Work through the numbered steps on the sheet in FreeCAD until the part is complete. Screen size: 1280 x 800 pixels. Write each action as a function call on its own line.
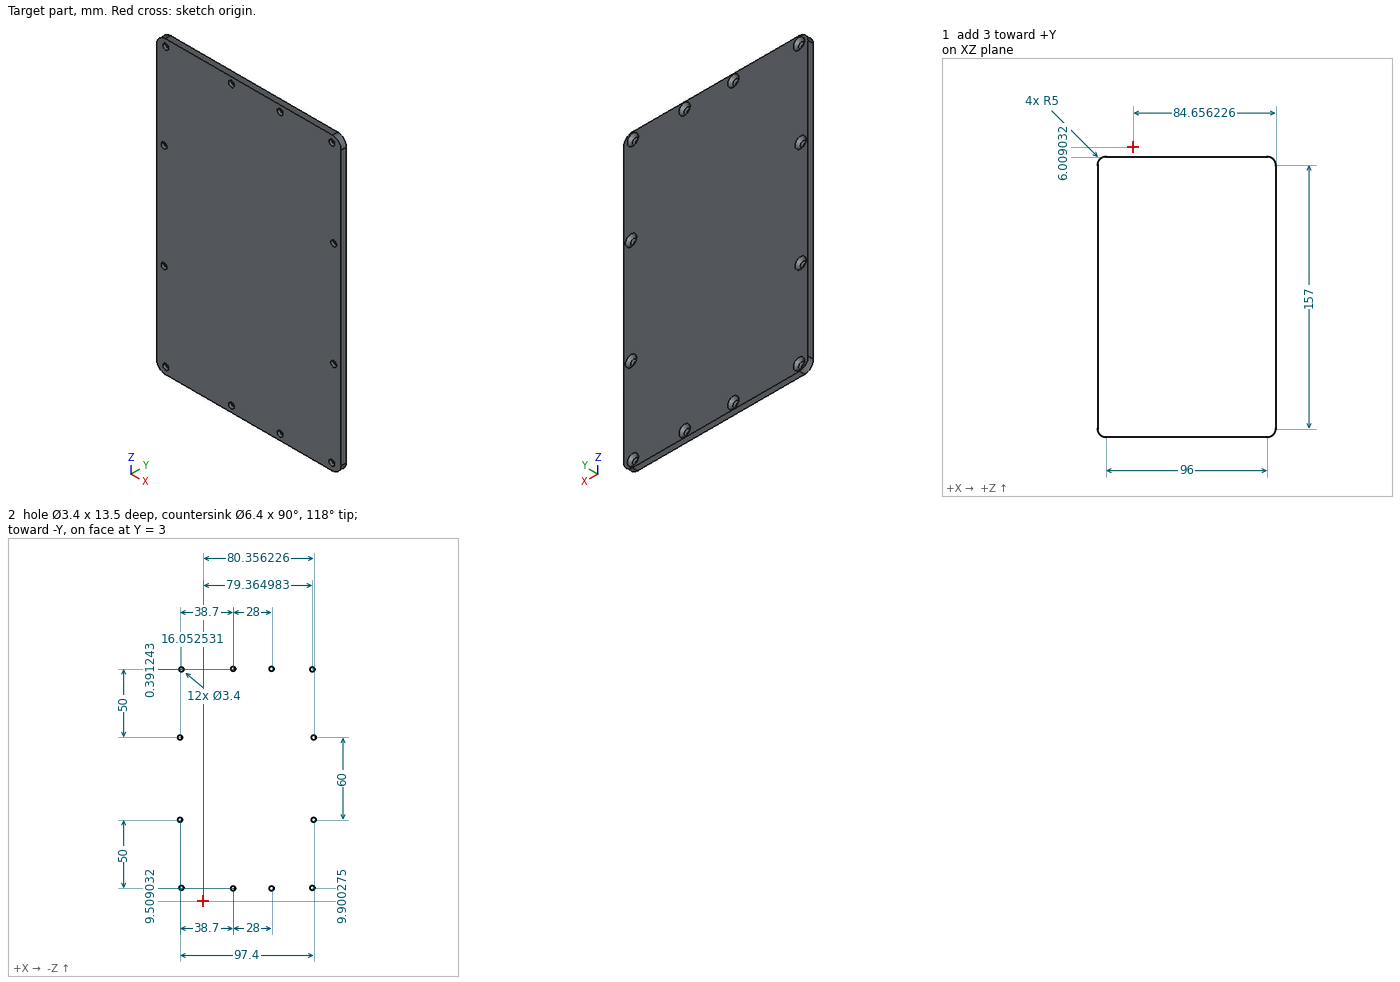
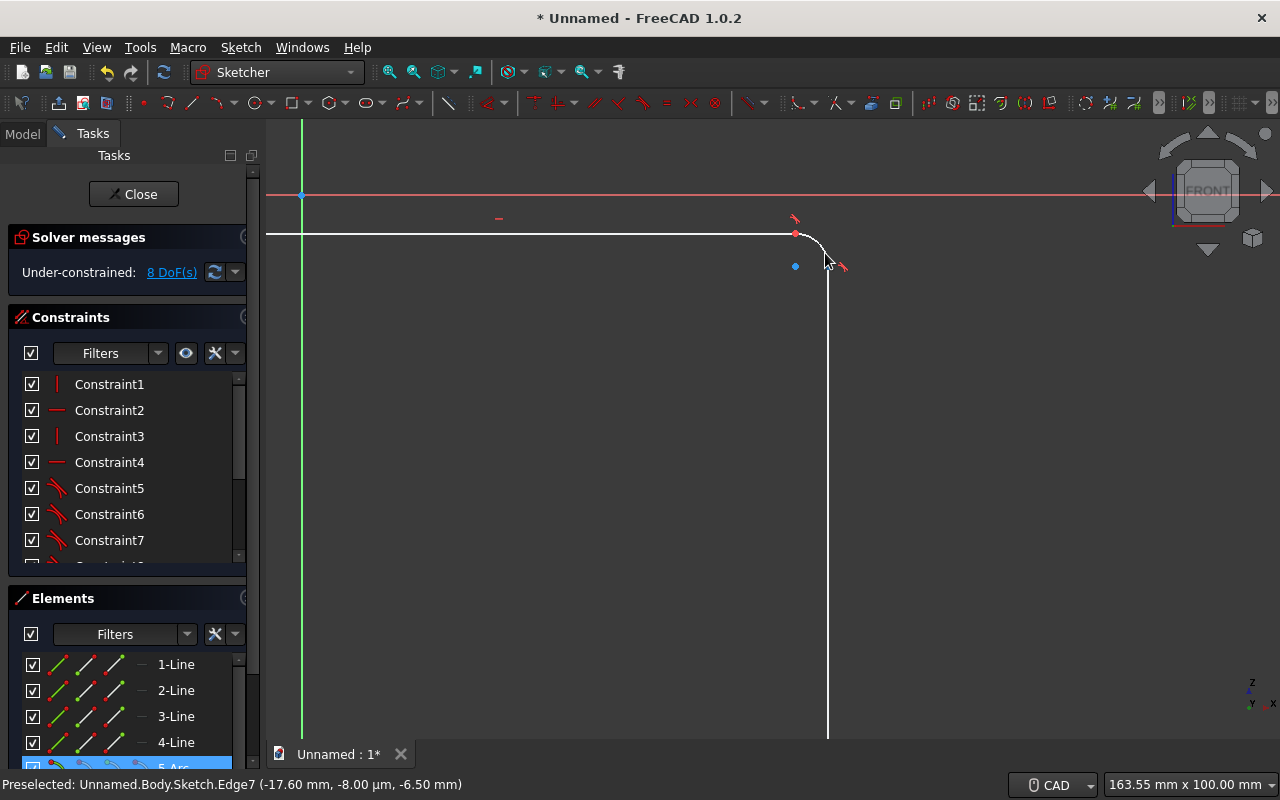
click(825, 252)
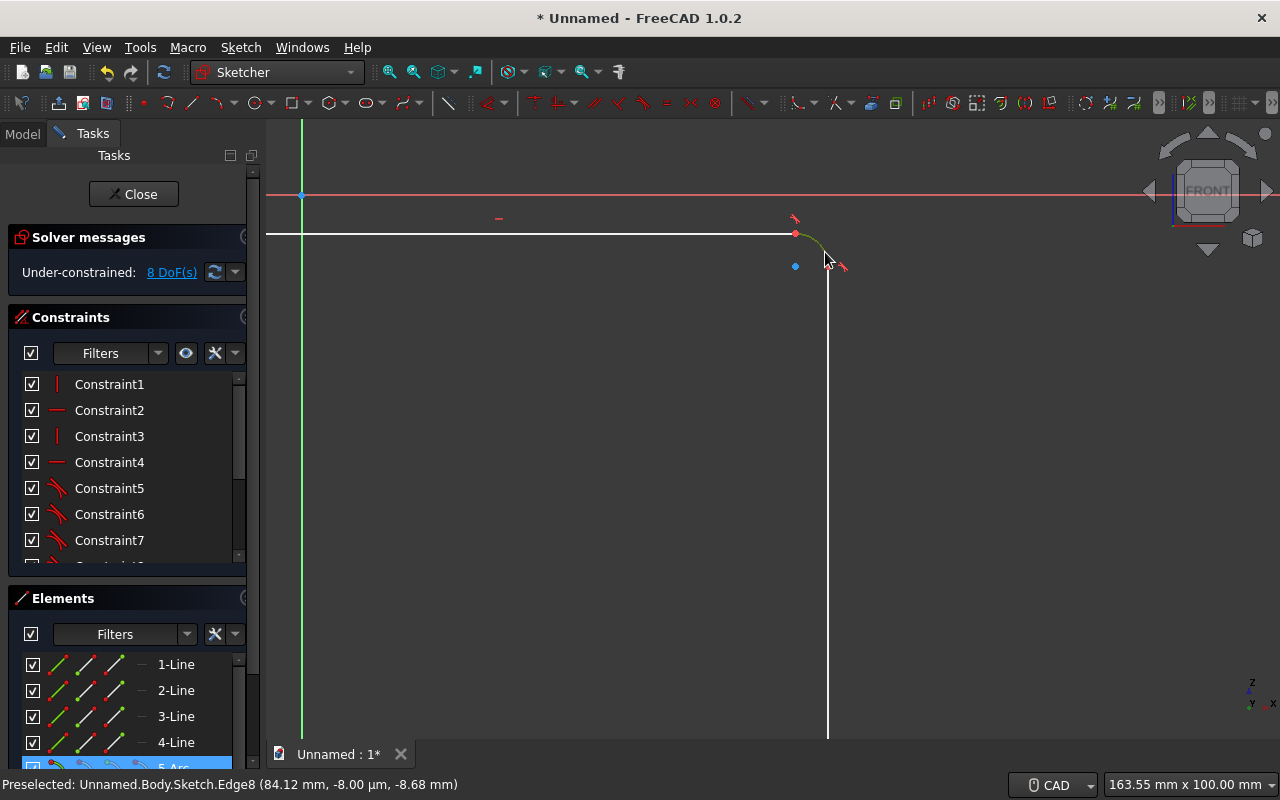
click(668, 104)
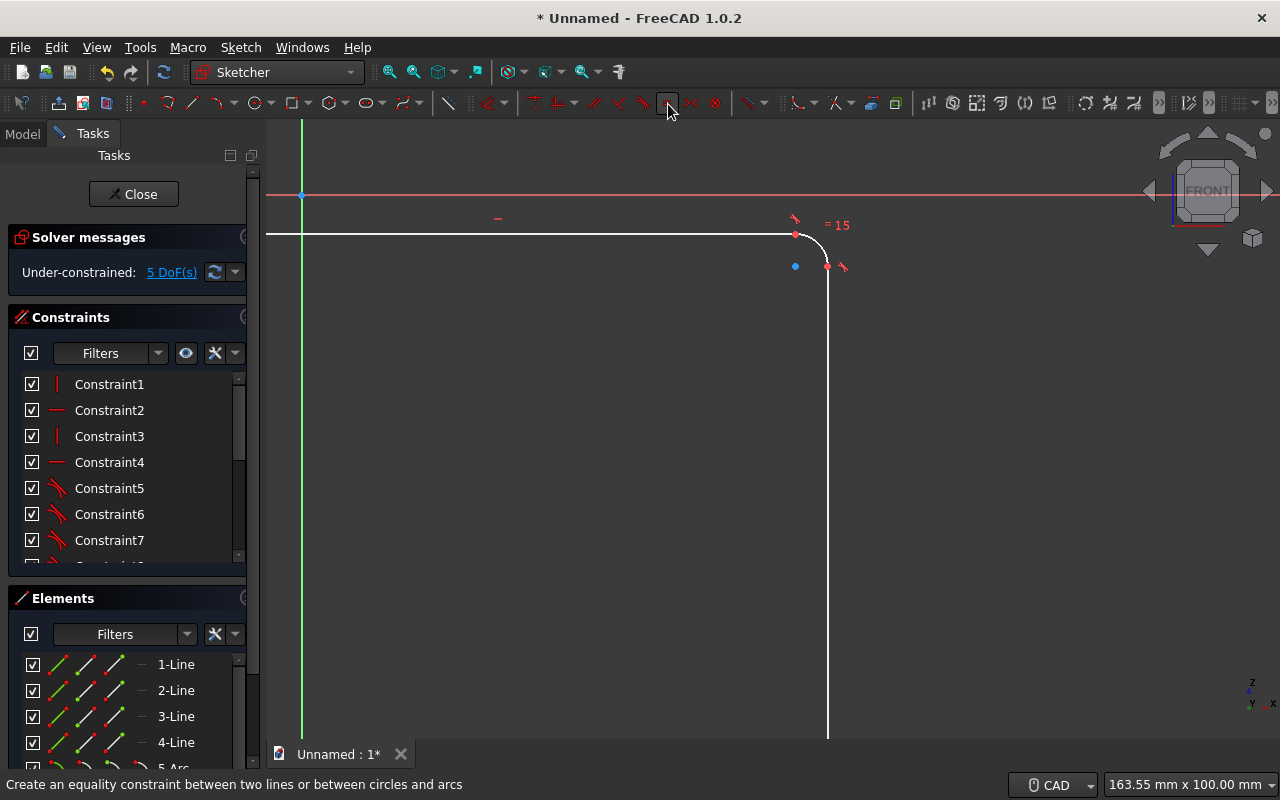
click(488, 104)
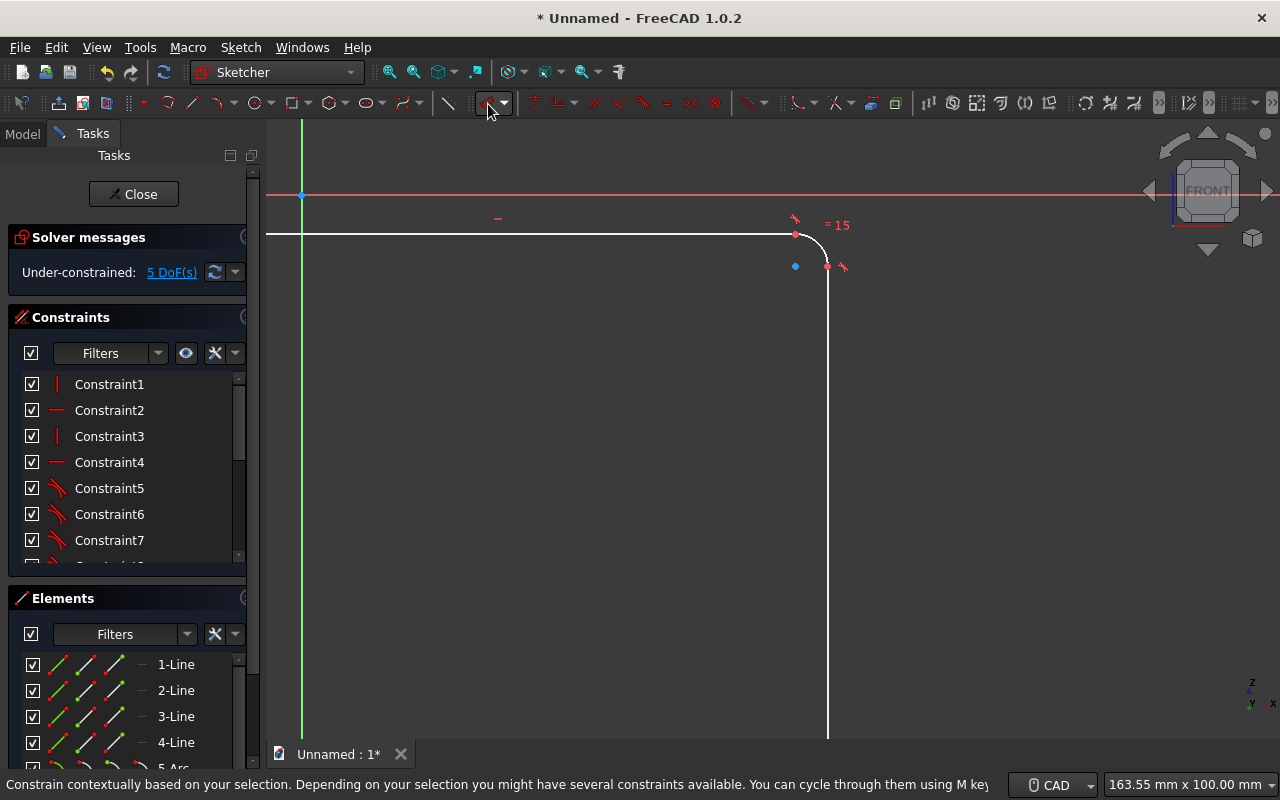
scroll(825, 253, down, 5)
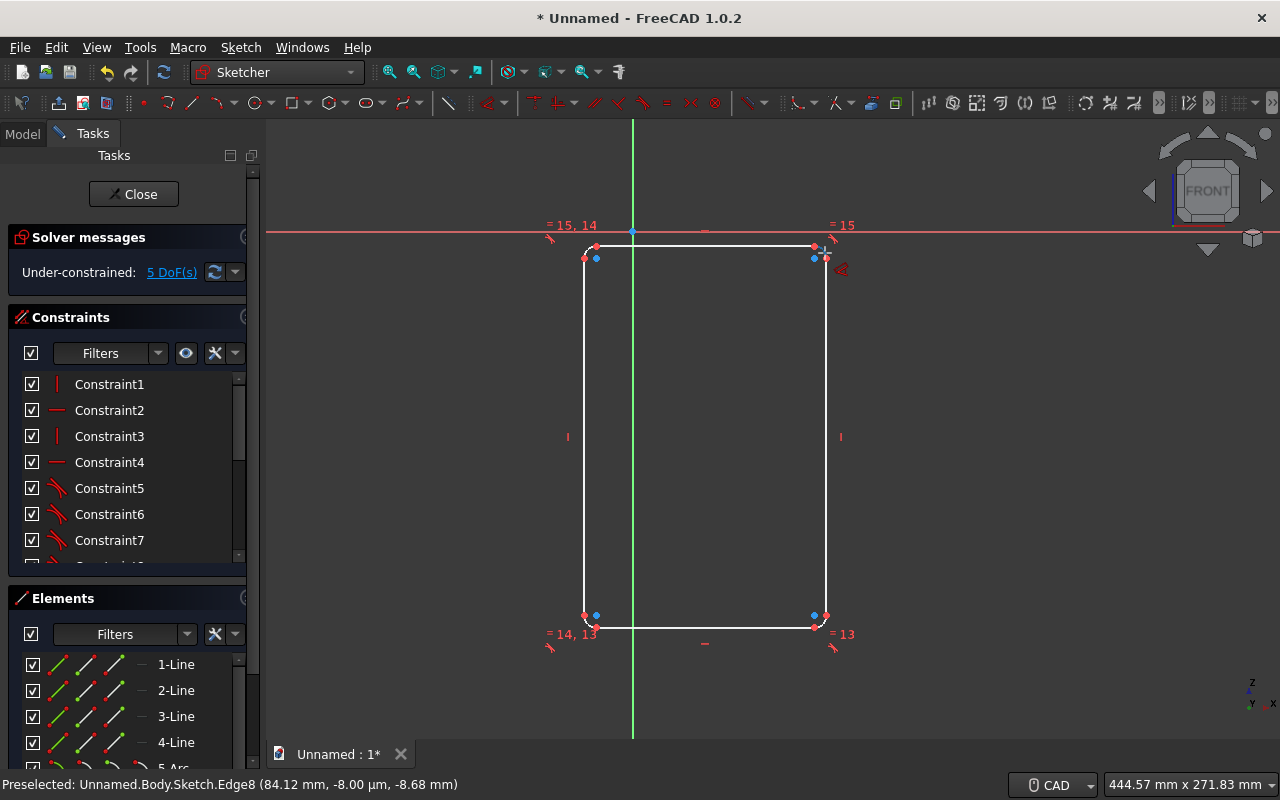
scroll(820, 627, up, 7)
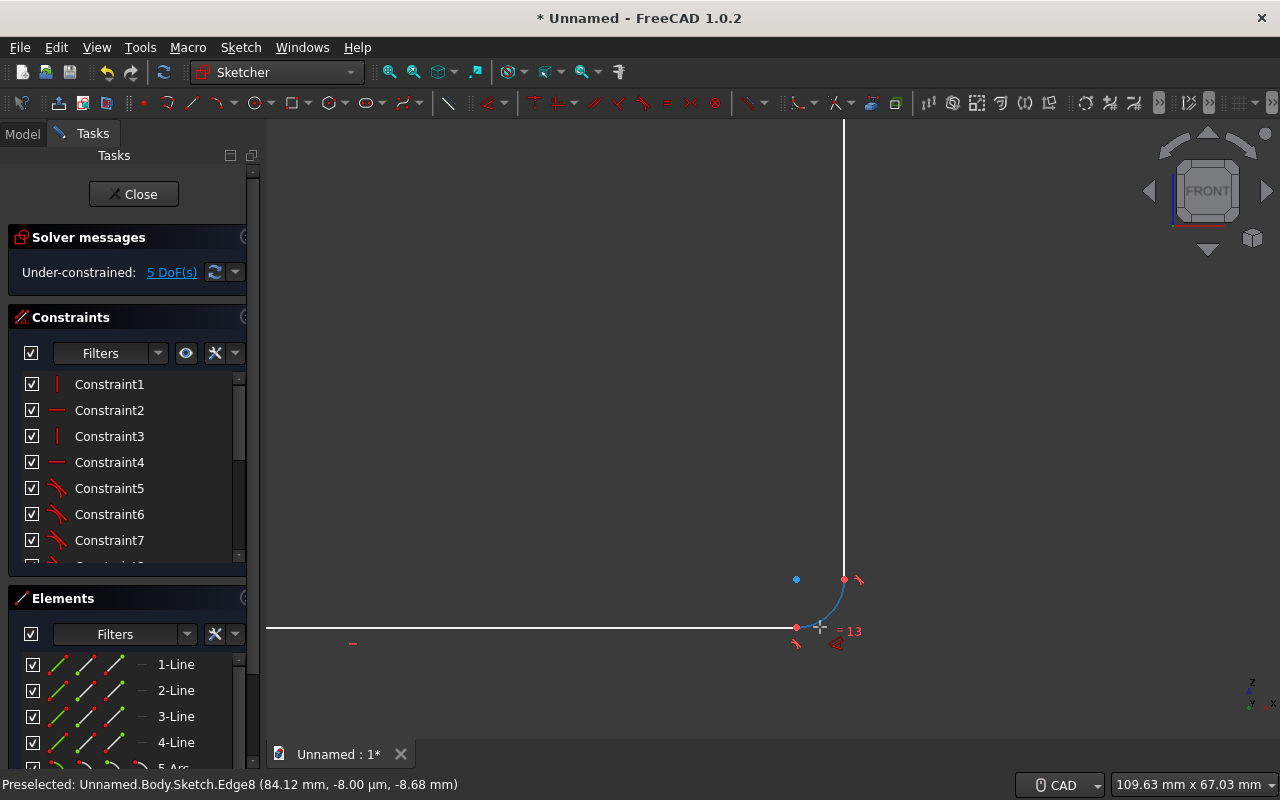
click(818, 623)
click(832, 652)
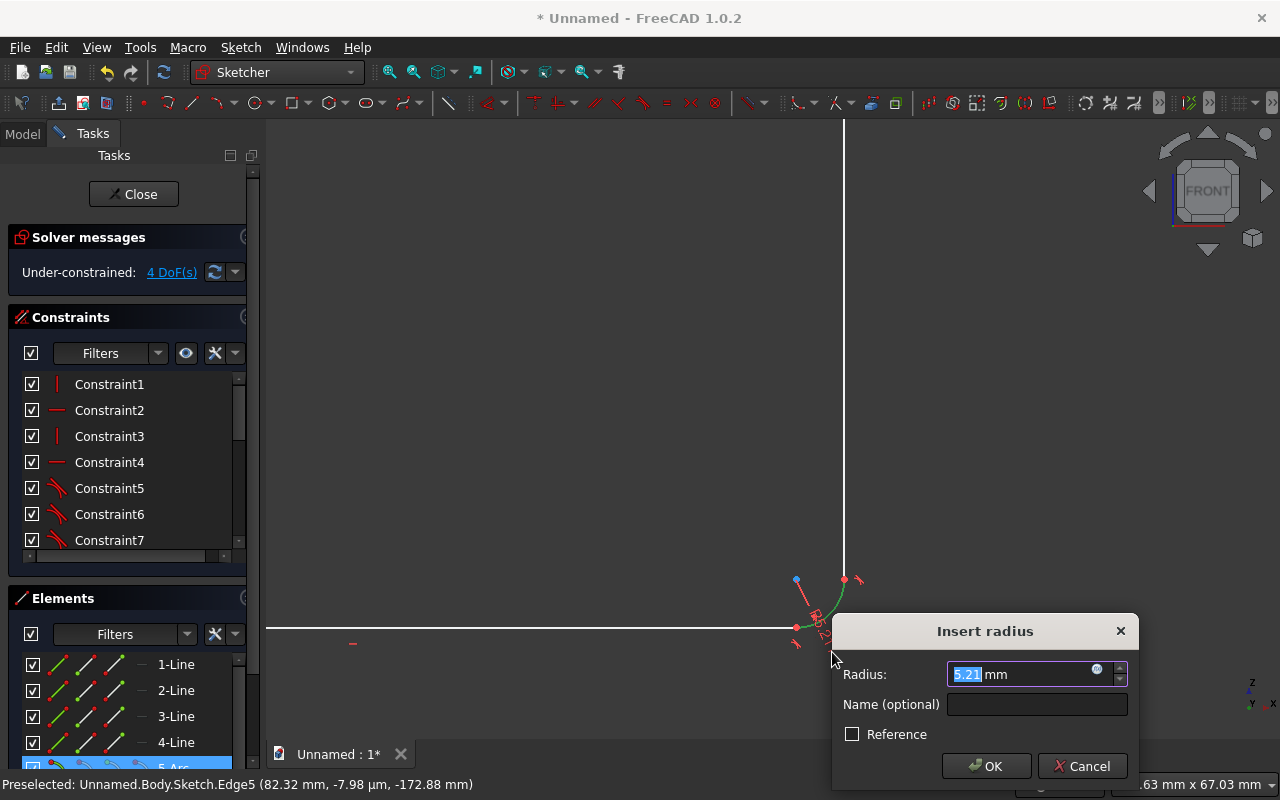
text(5)
key(Return)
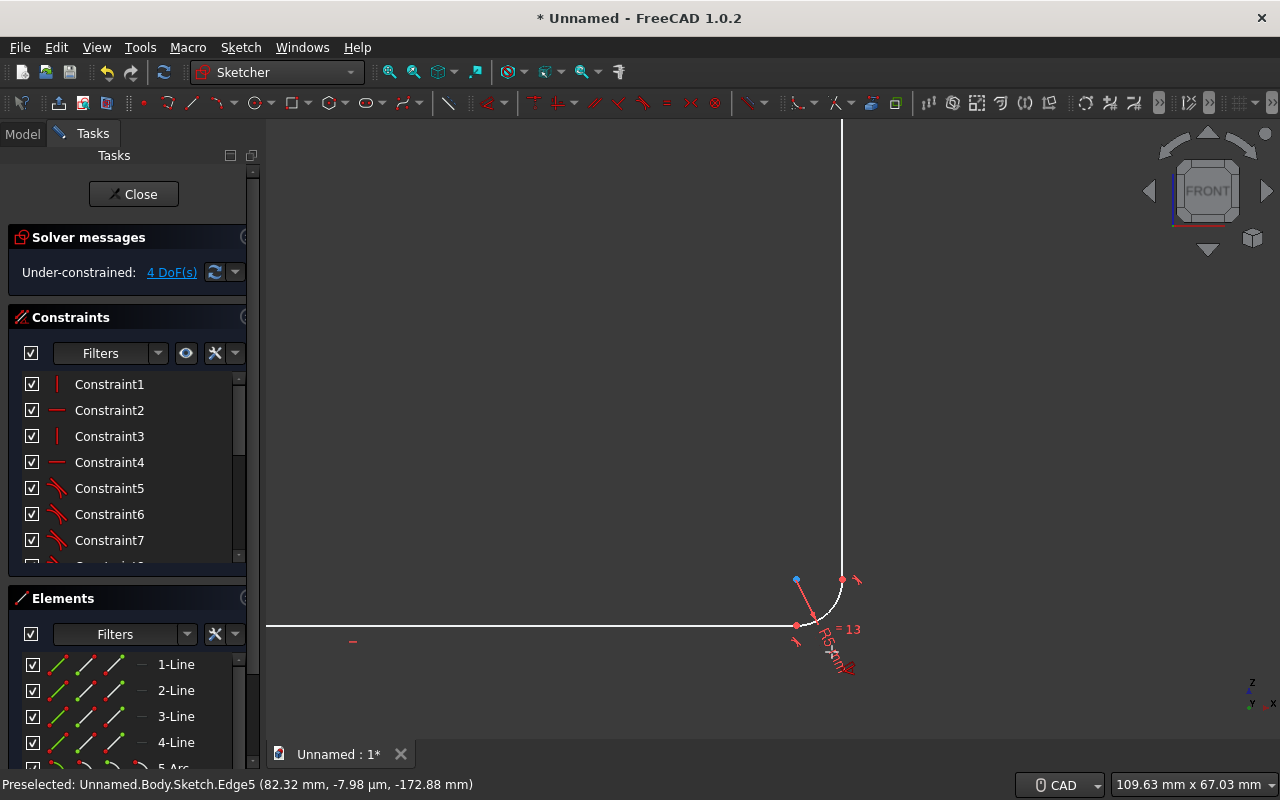
scroll(820, 628, down, 7)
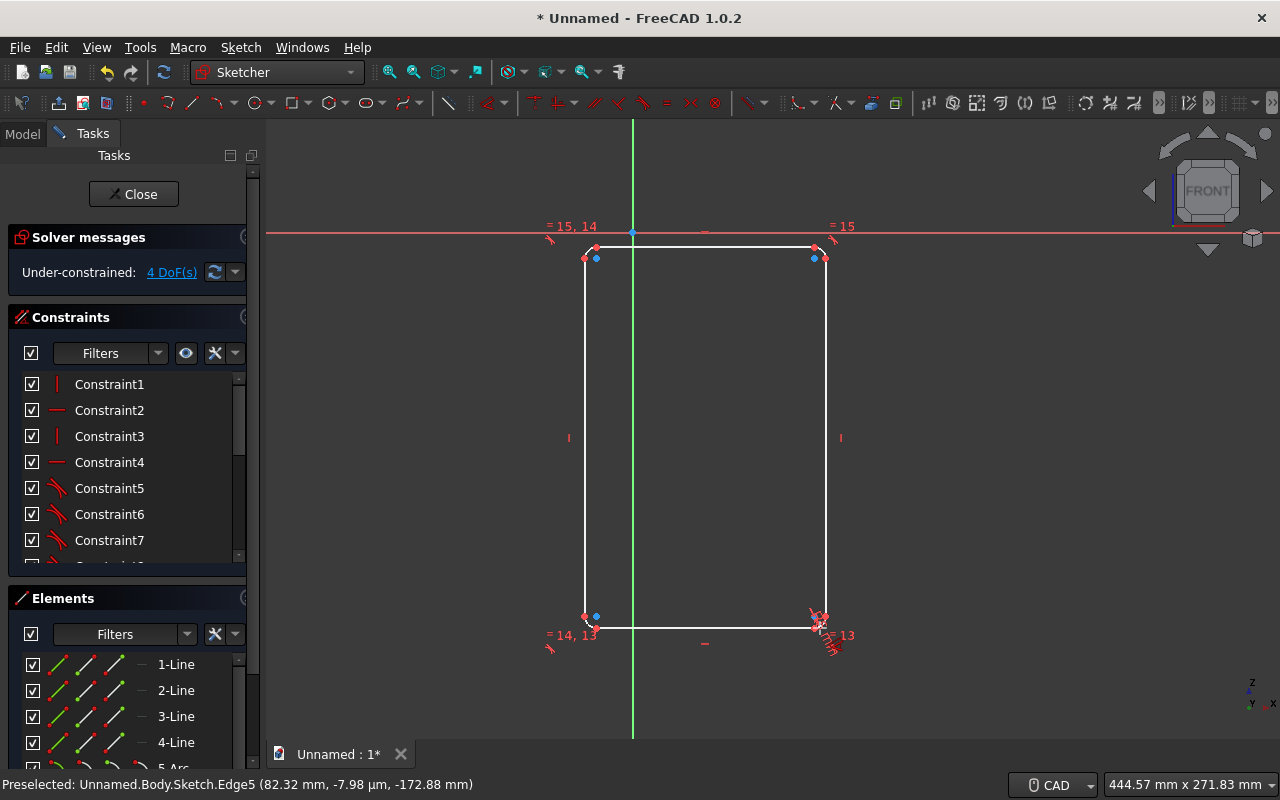
click(749, 628)
click(705, 662)